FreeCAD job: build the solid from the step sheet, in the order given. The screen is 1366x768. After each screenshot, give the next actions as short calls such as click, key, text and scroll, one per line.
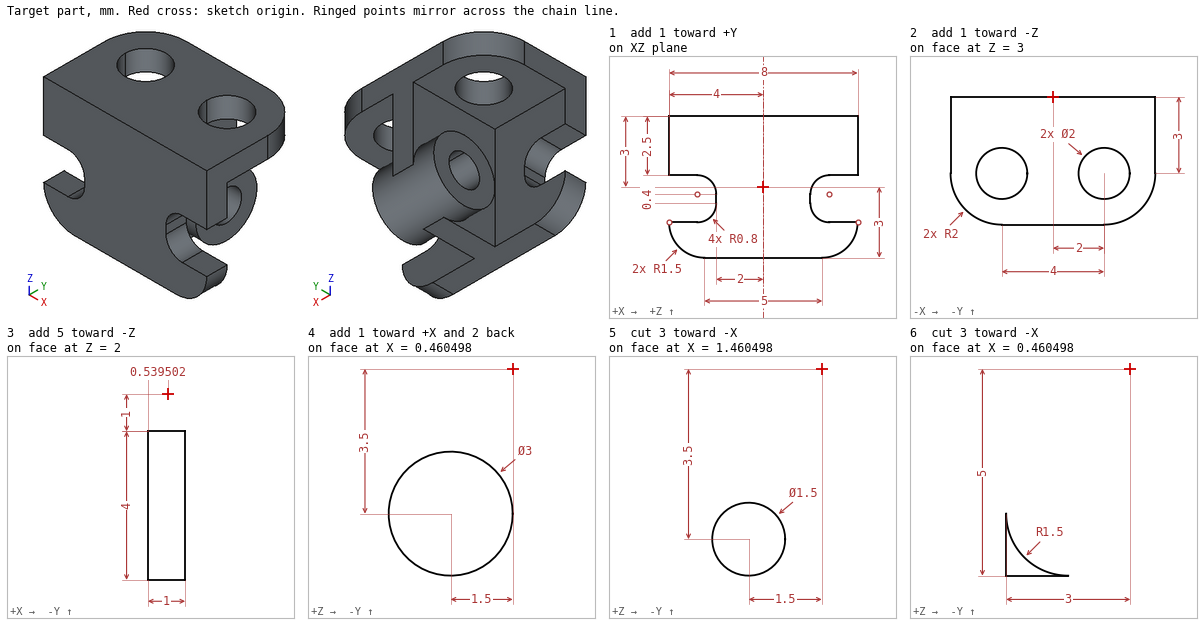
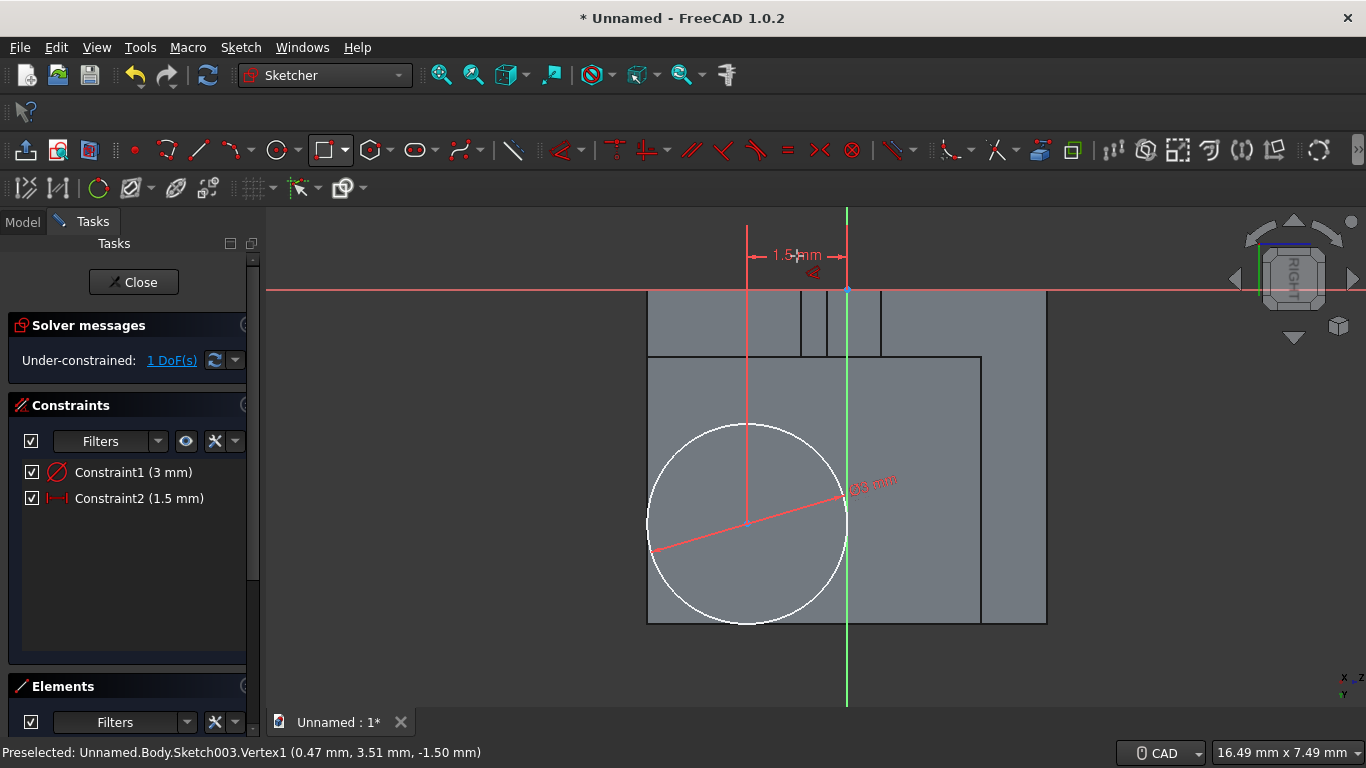
click(747, 524)
click(881, 407)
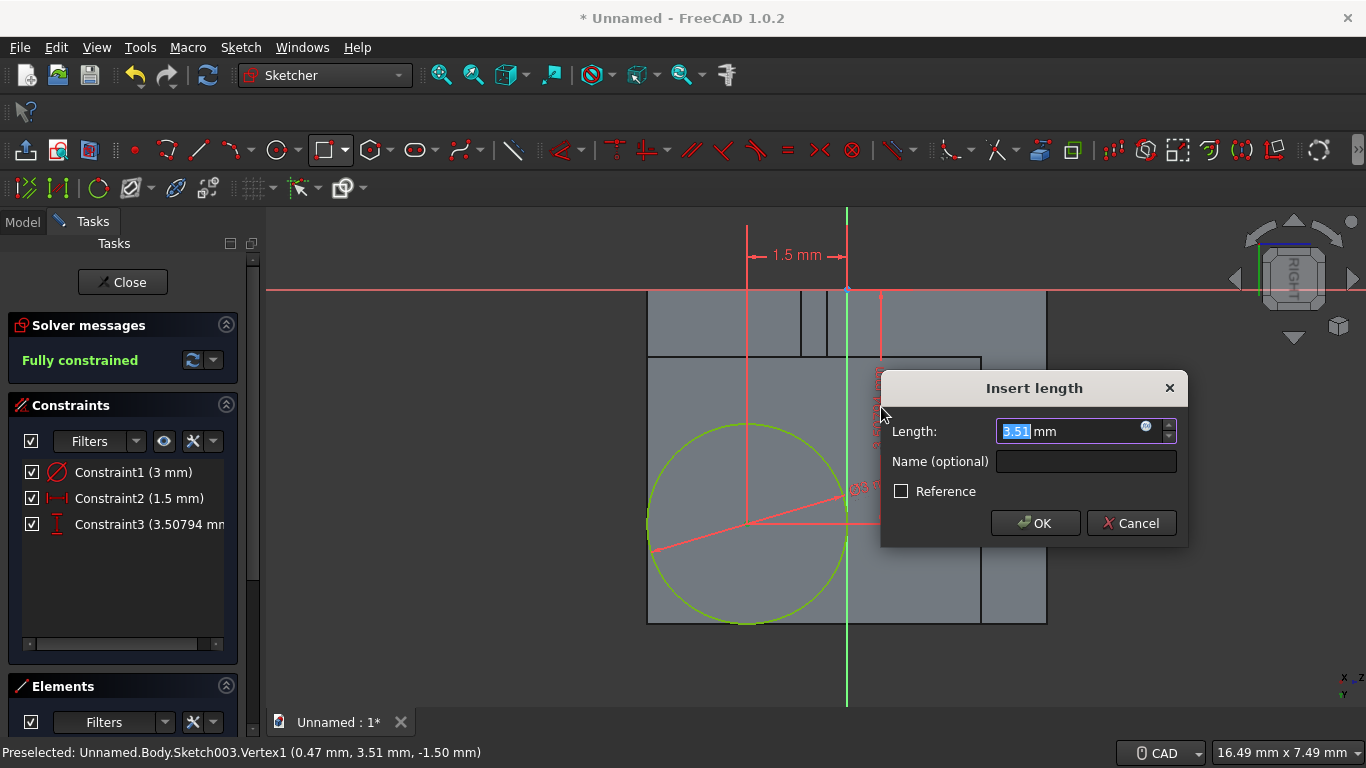
text(3.5)
key(Return)
key(Escape)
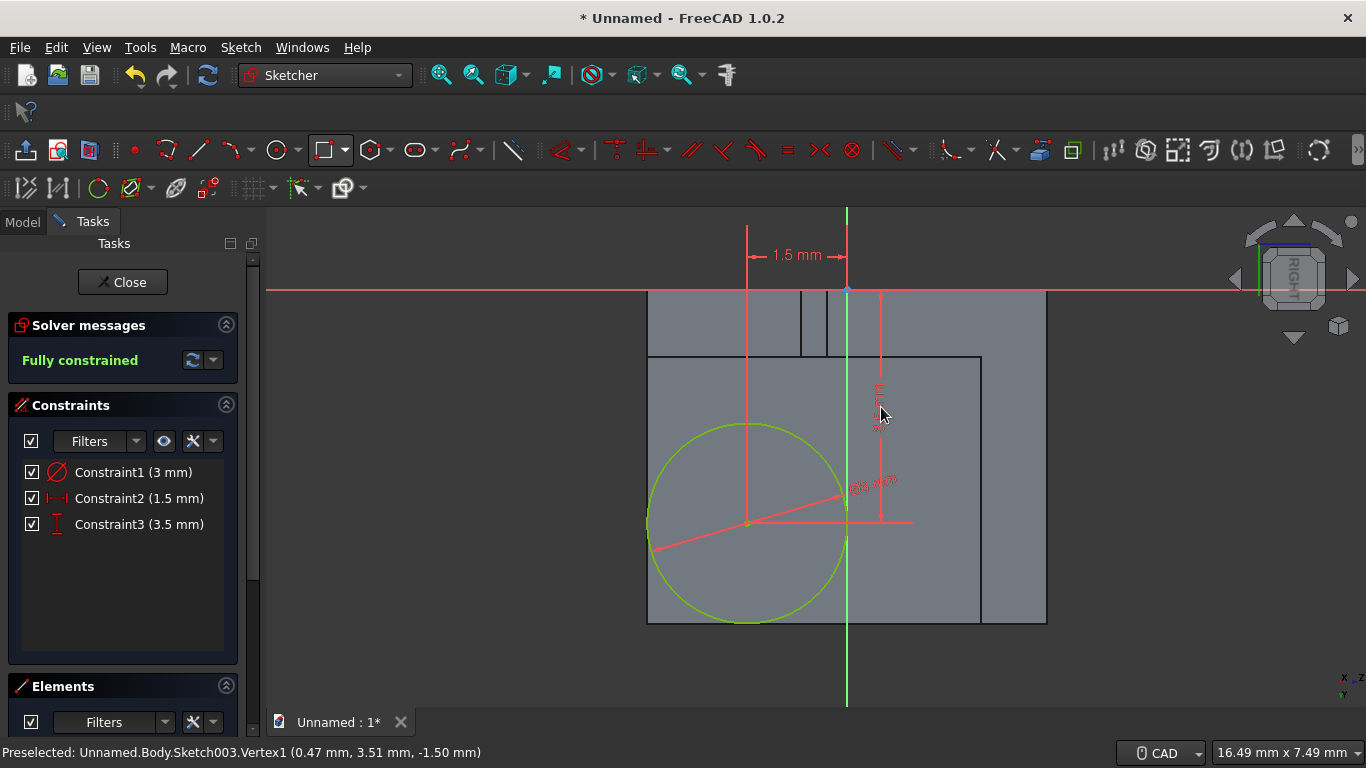
click(123, 282)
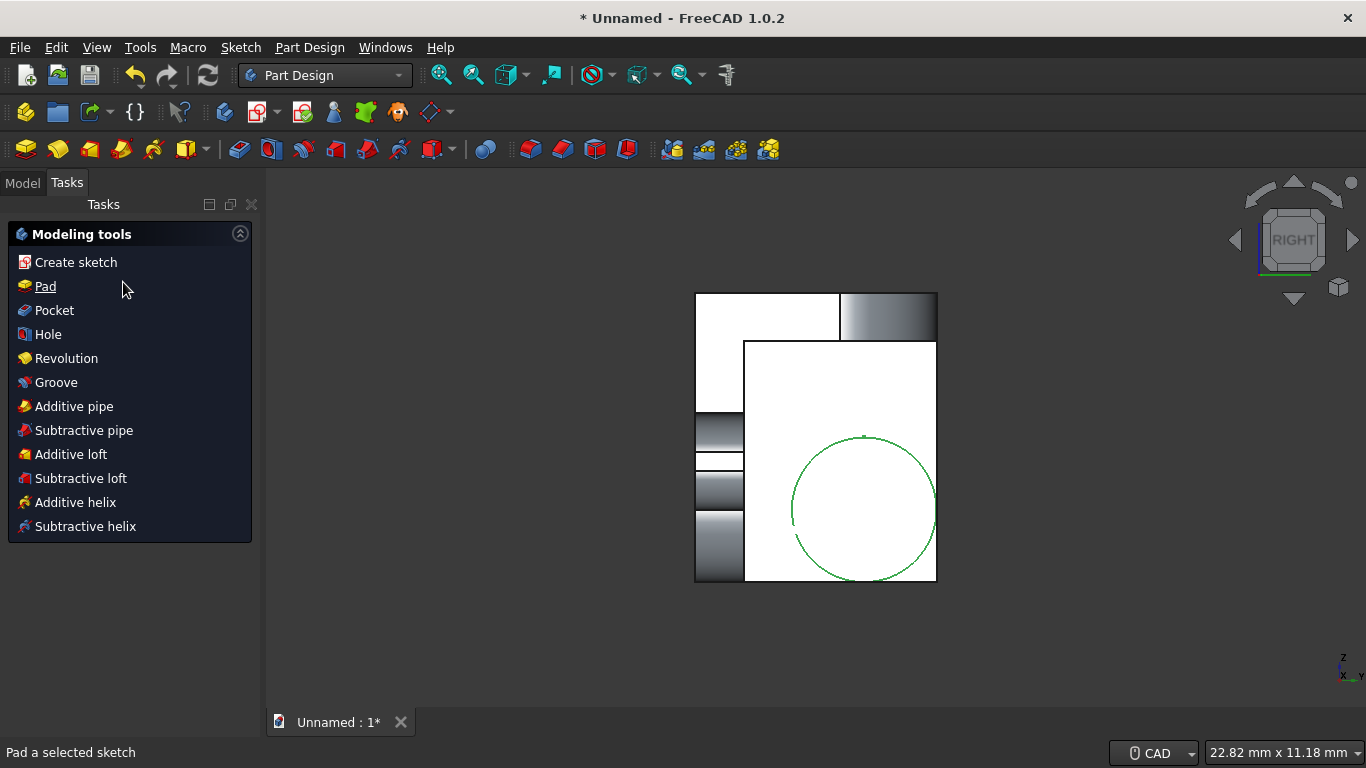
click(26, 150)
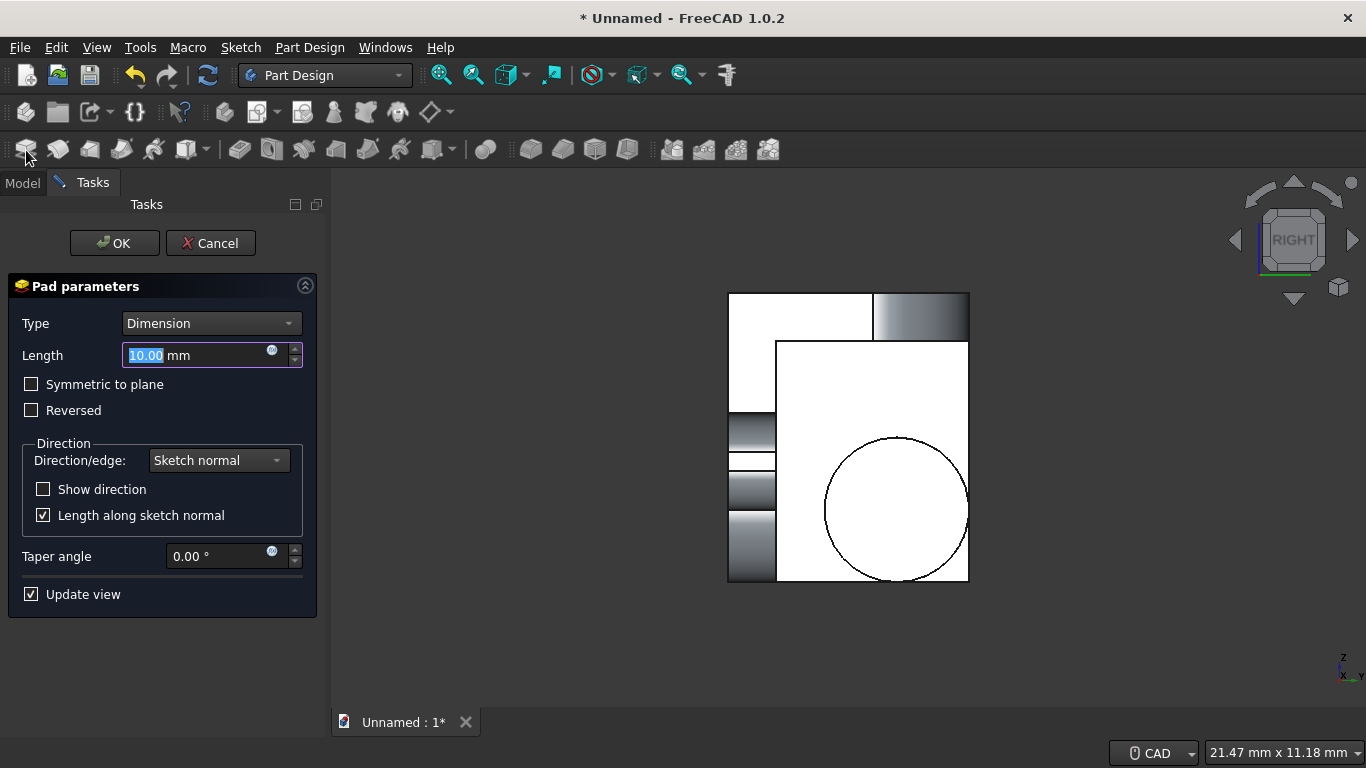
click(212, 324)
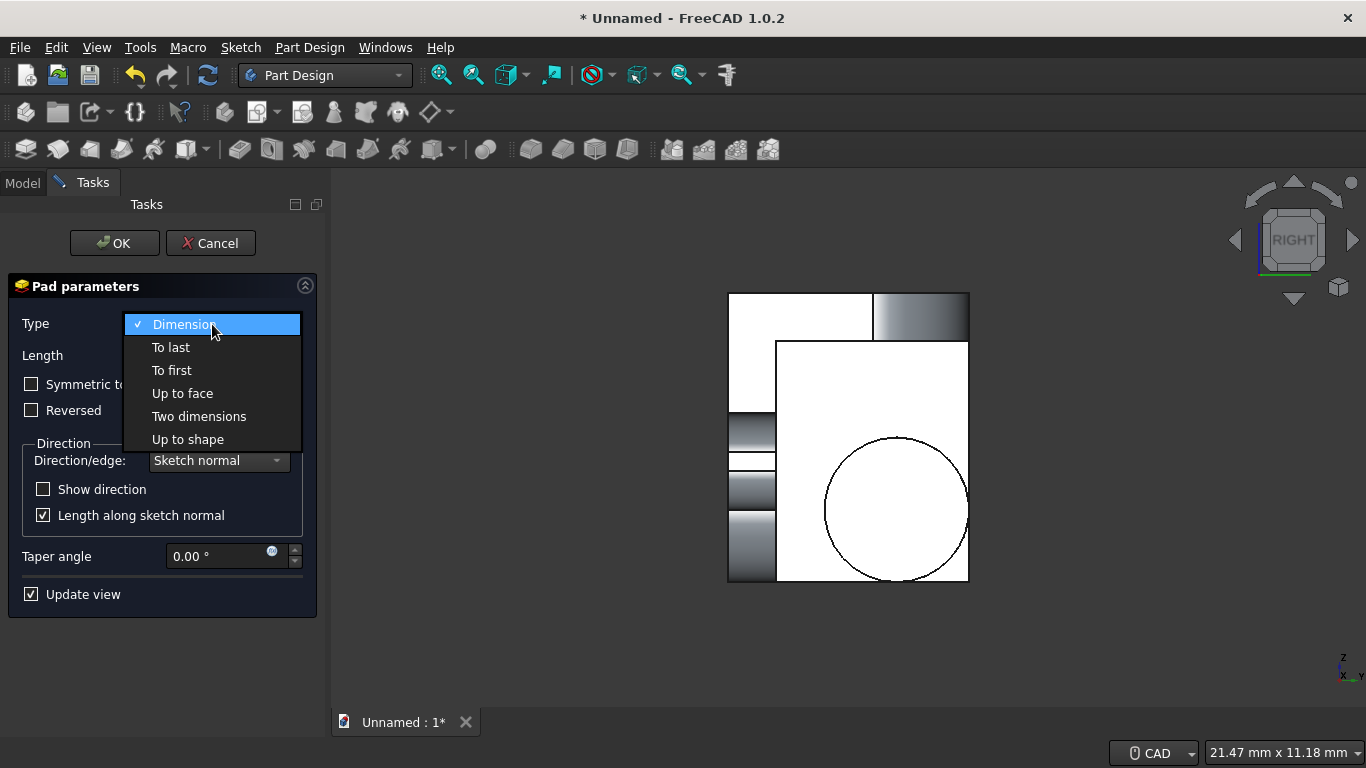
click(212, 416)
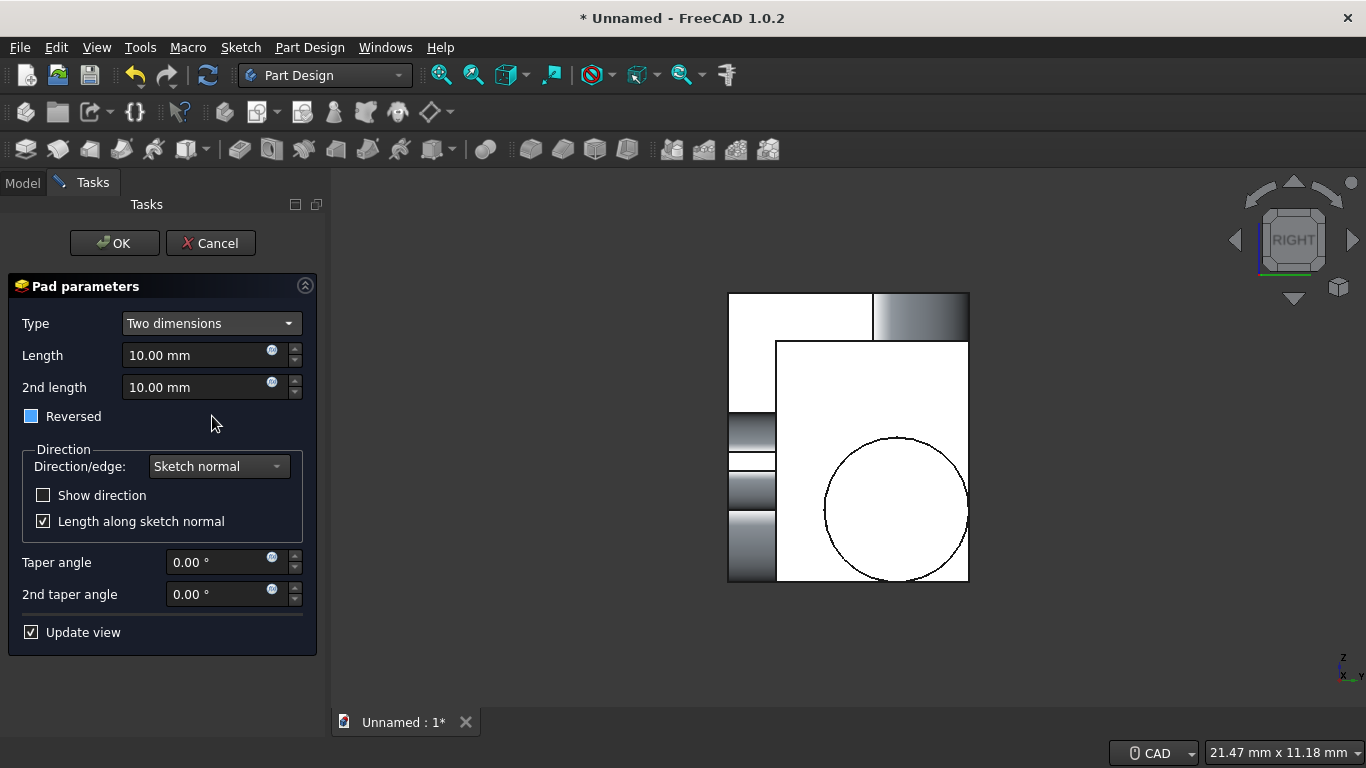
triple_click(204, 355)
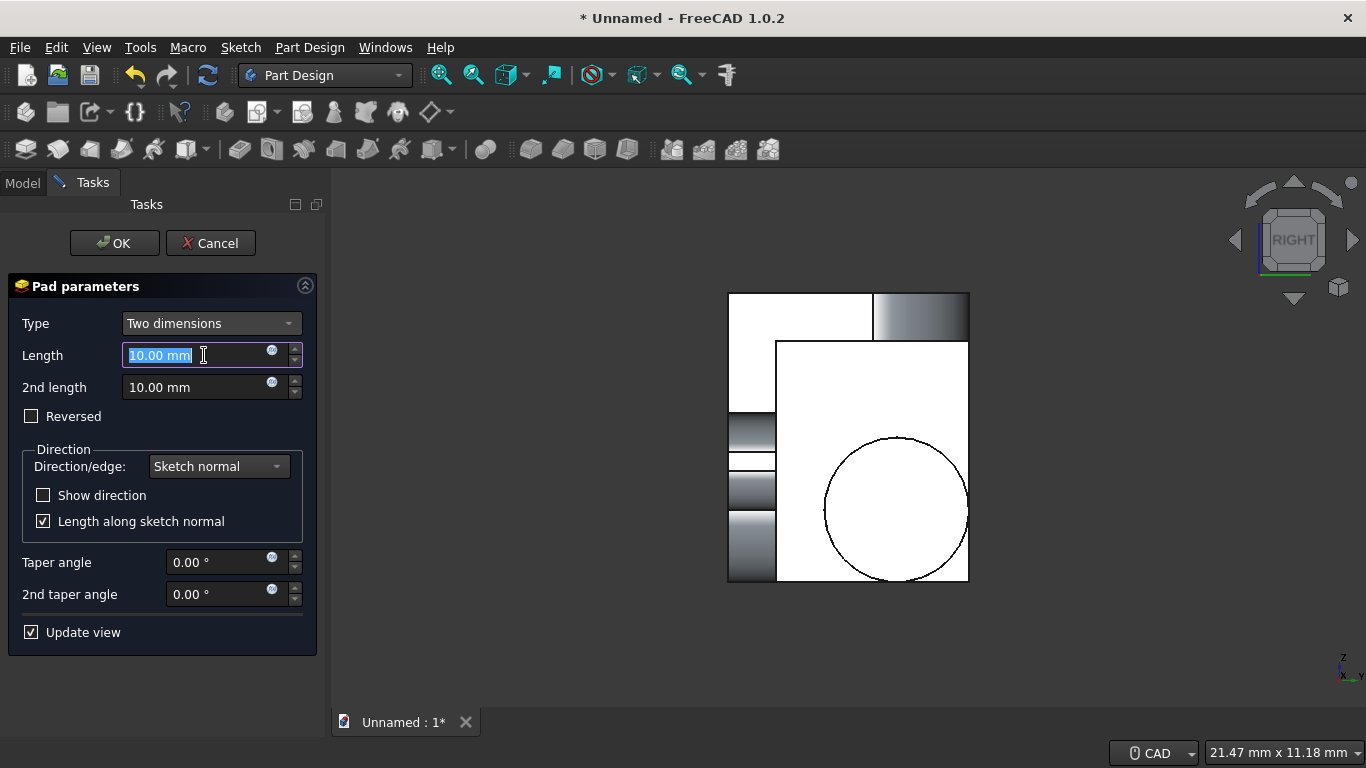
text(1)
key(Tab)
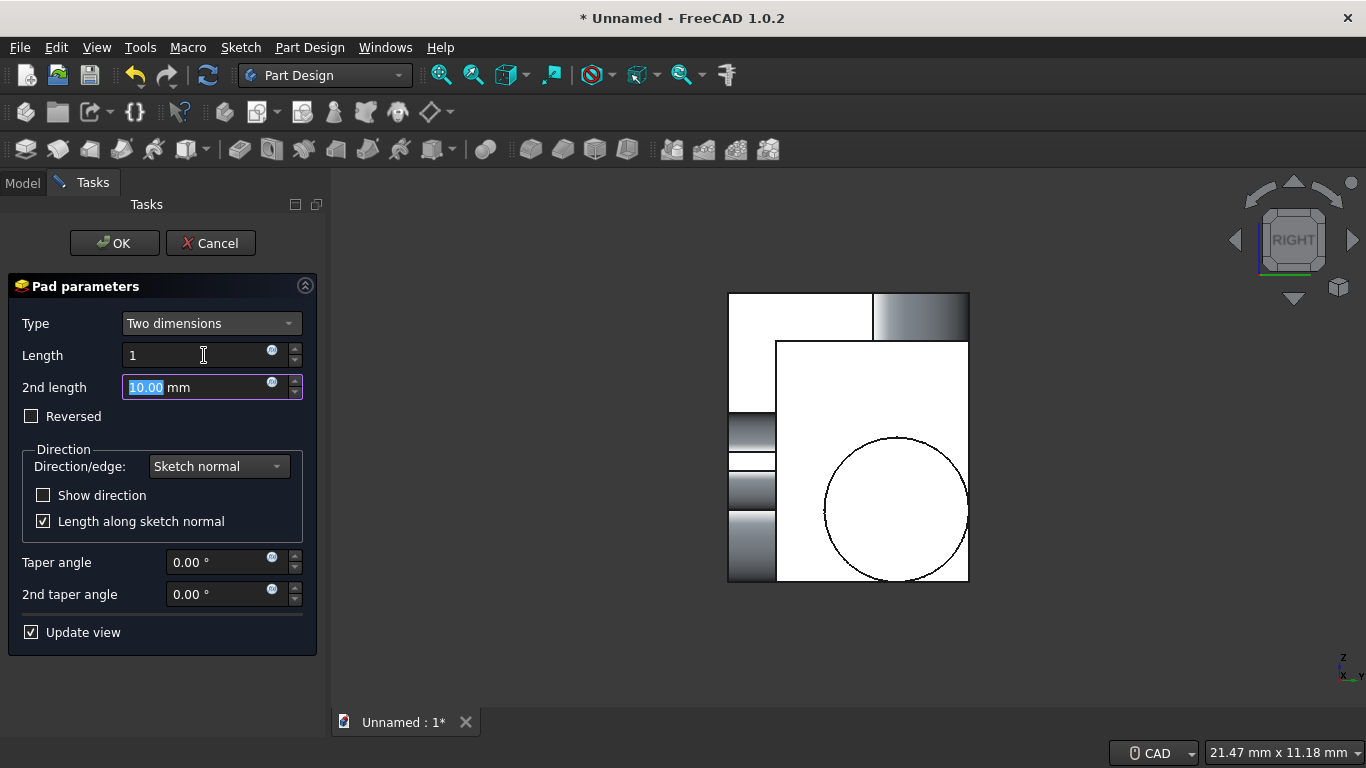
text(2)
key(Tab)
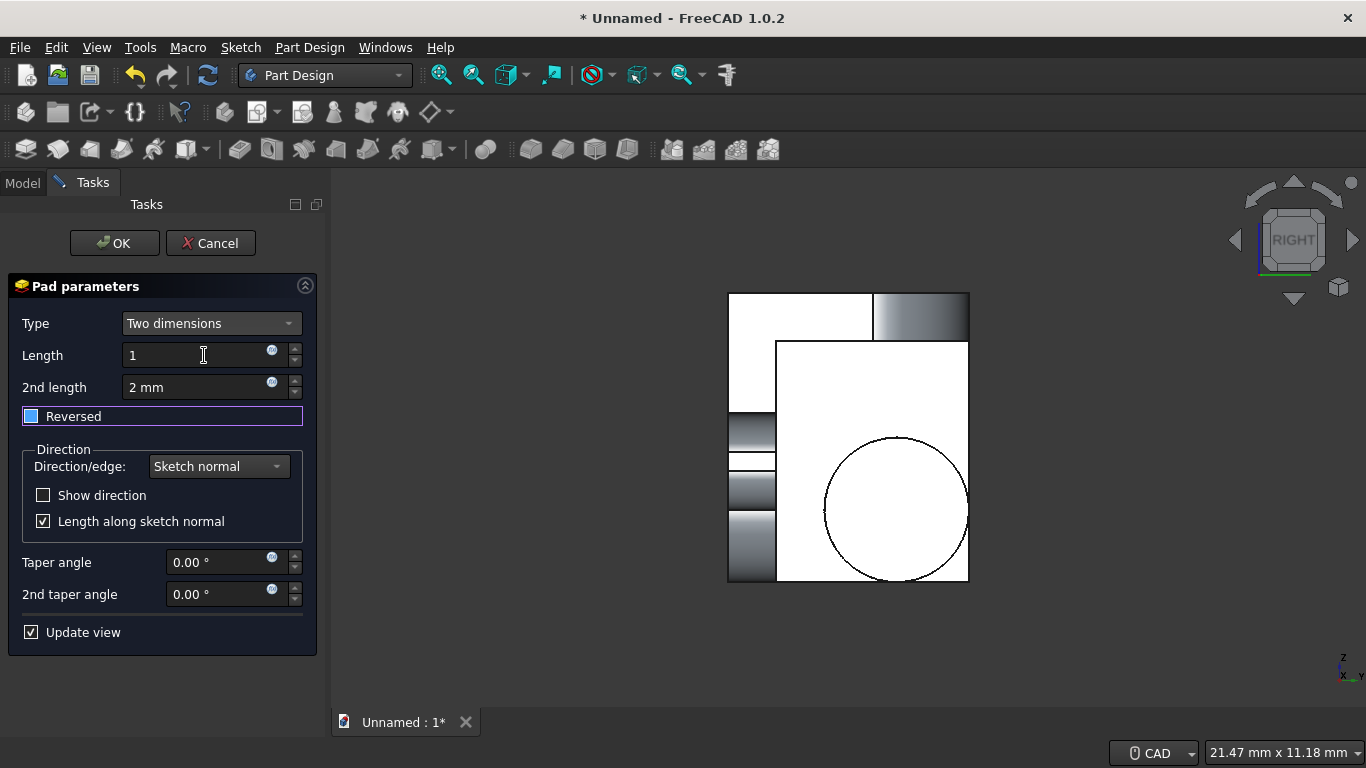
click(115, 243)